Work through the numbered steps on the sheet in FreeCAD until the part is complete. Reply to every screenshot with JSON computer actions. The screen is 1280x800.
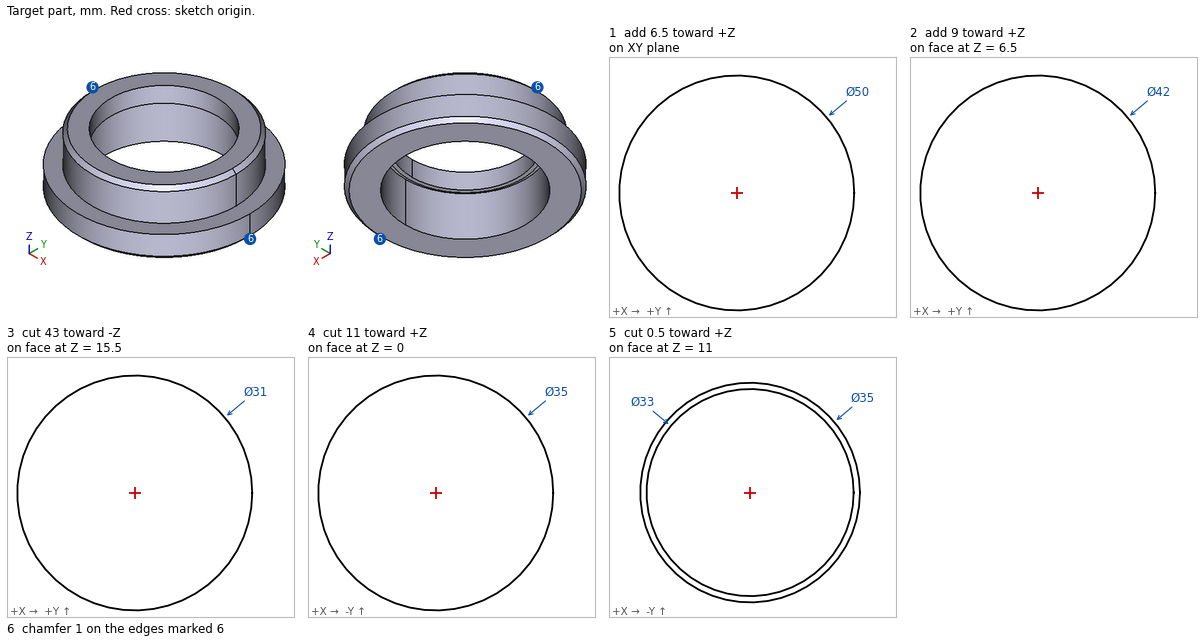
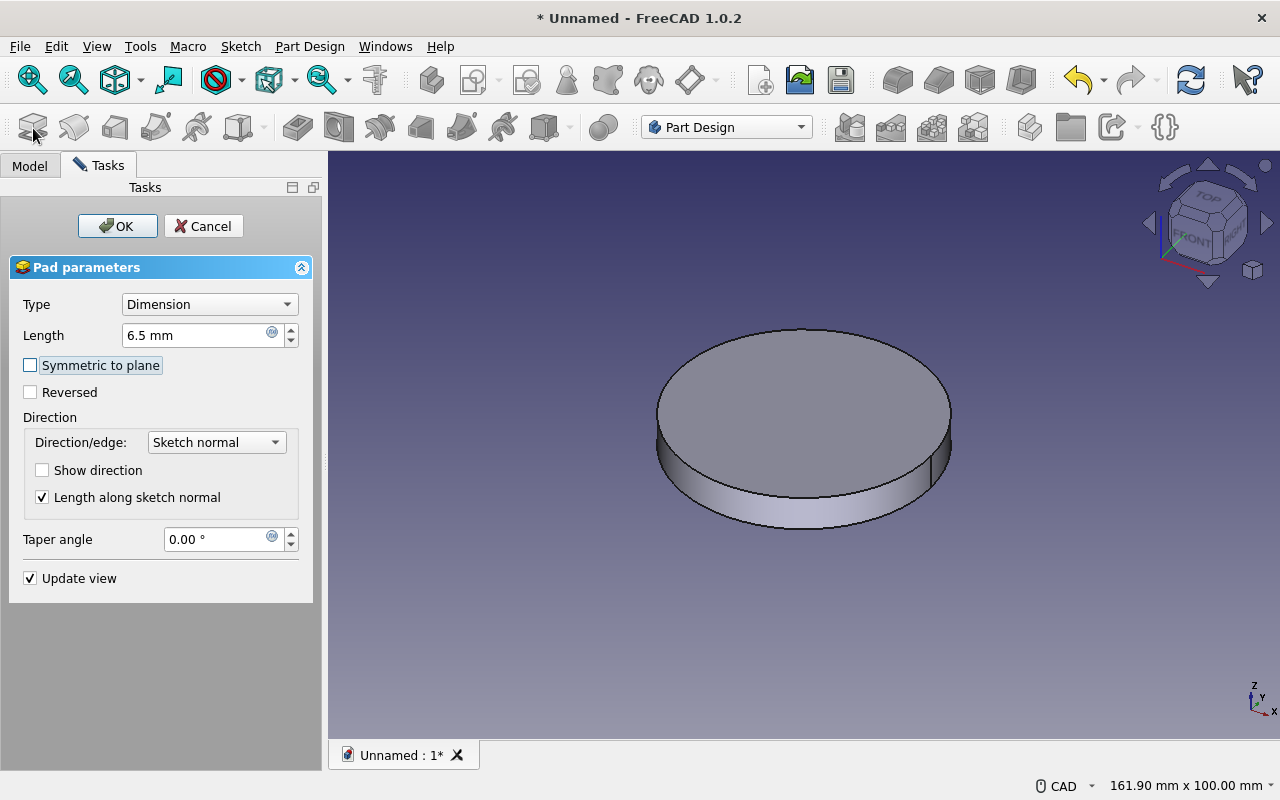
{"action": "left_click", "coordinate": [118, 226]}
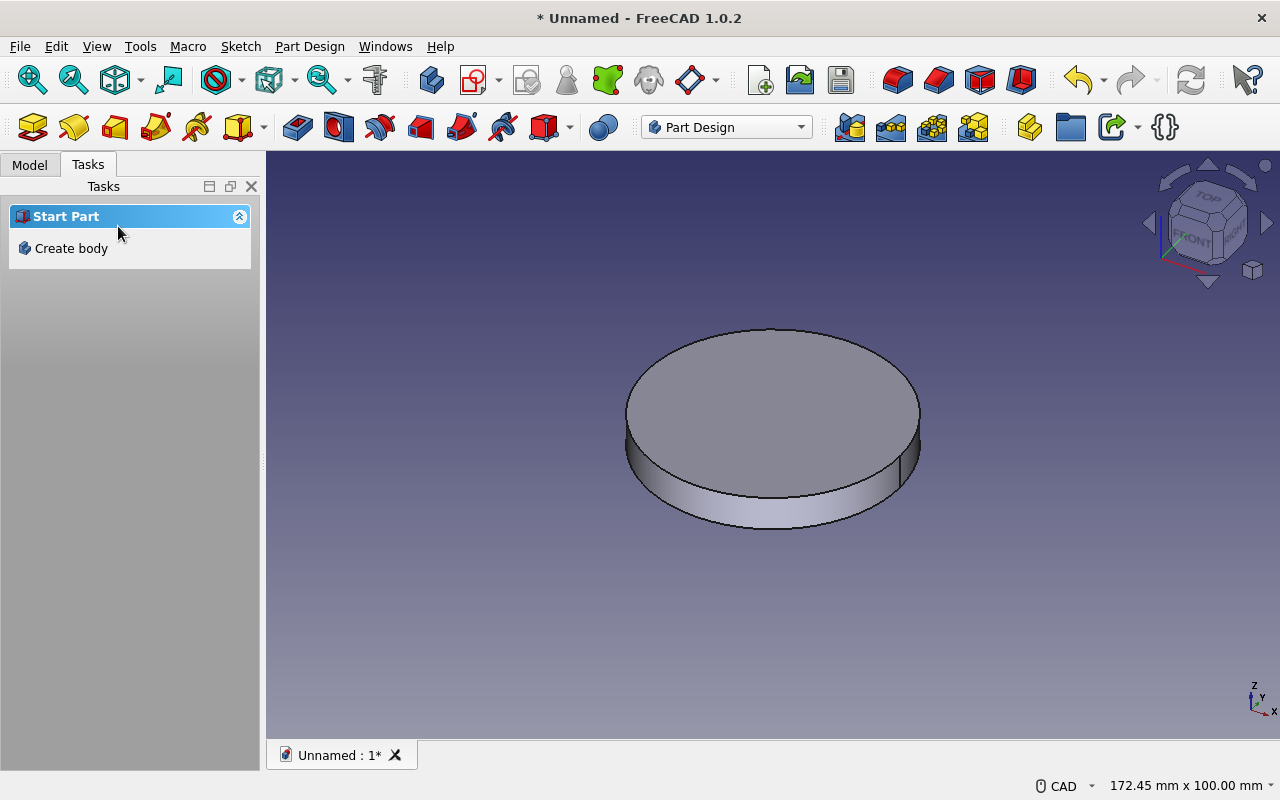
{"action": "left_click", "coordinate": [33, 80]}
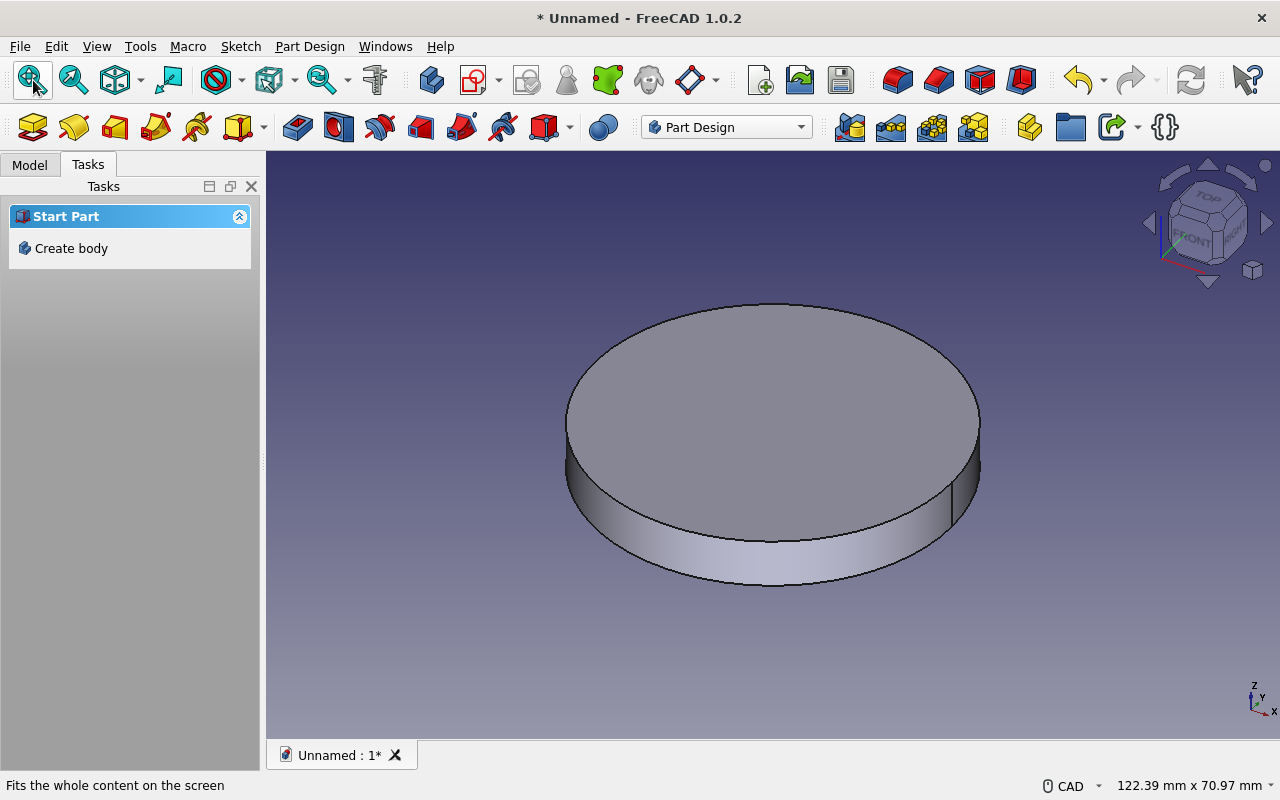
{"action": "left_click", "coordinate": [773, 422]}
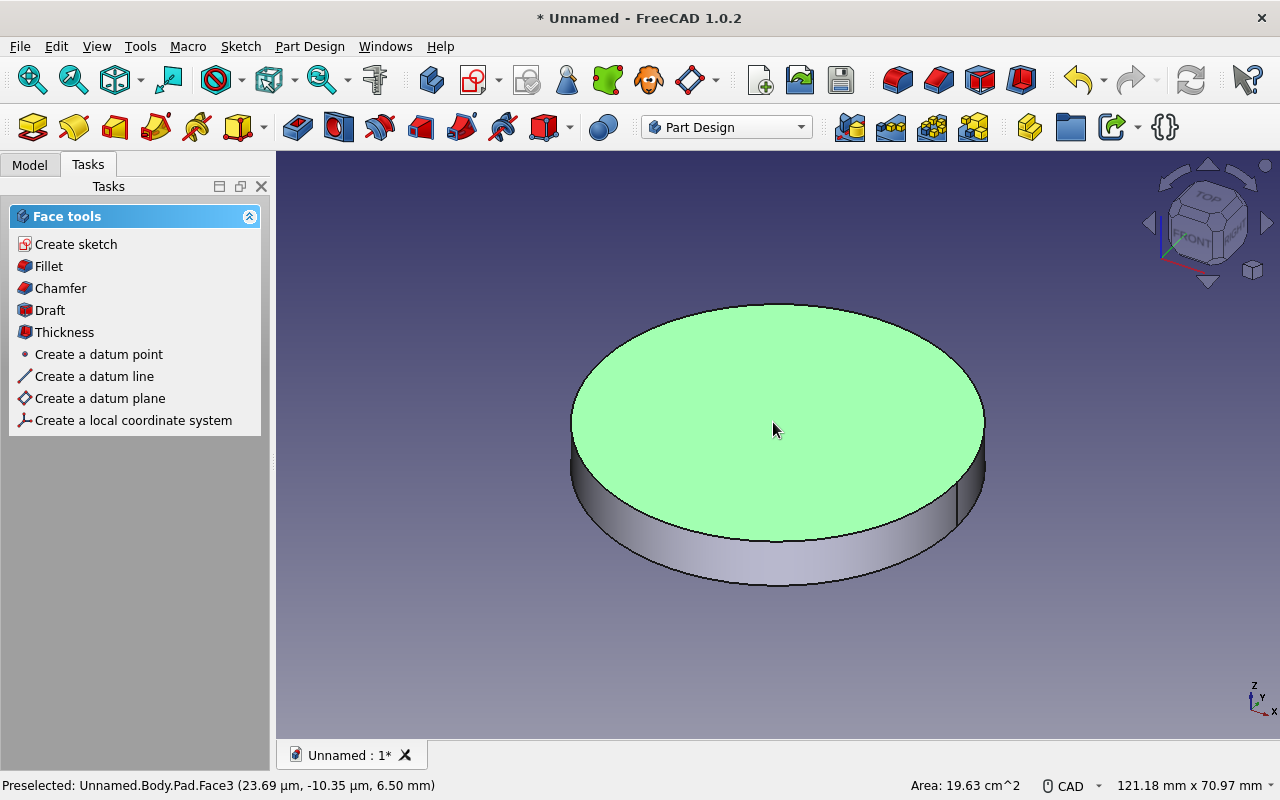
{"action": "left_click", "coordinate": [472, 80]}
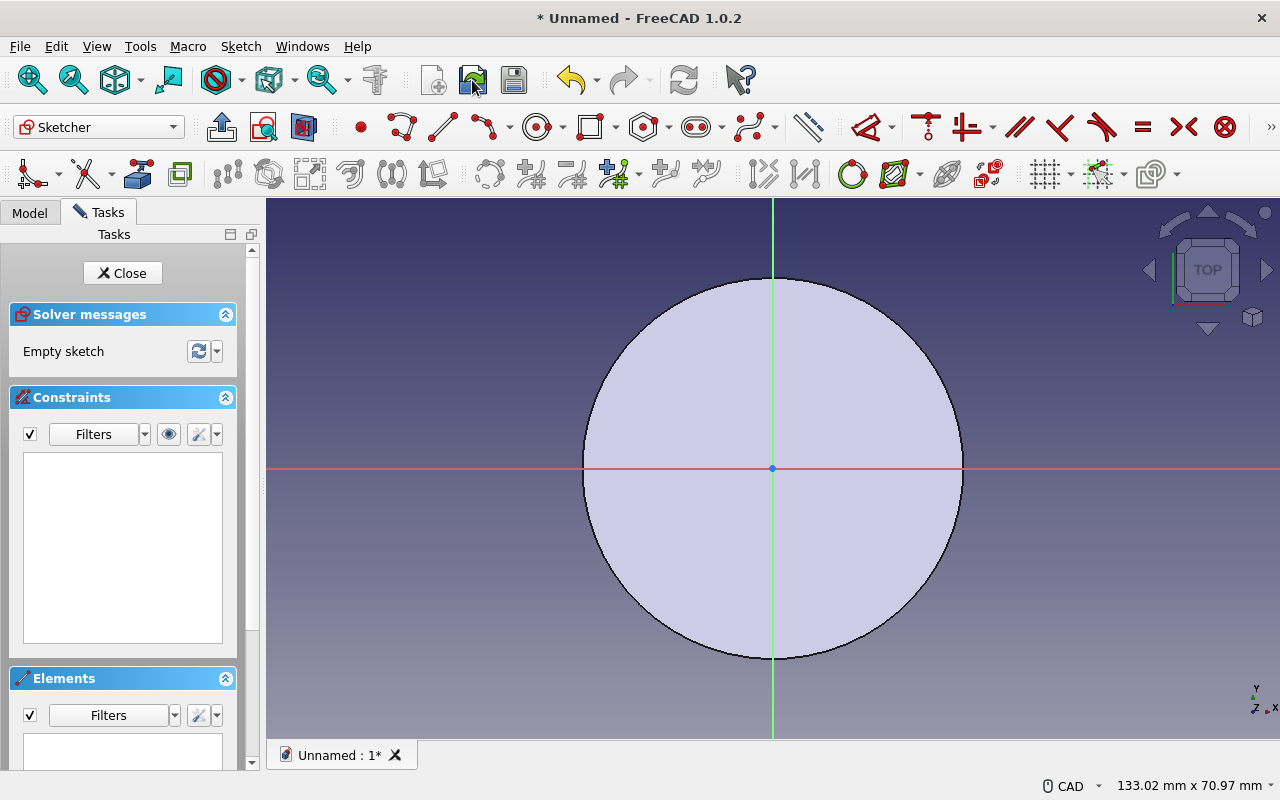
{"action": "left_click", "coordinate": [536, 128]}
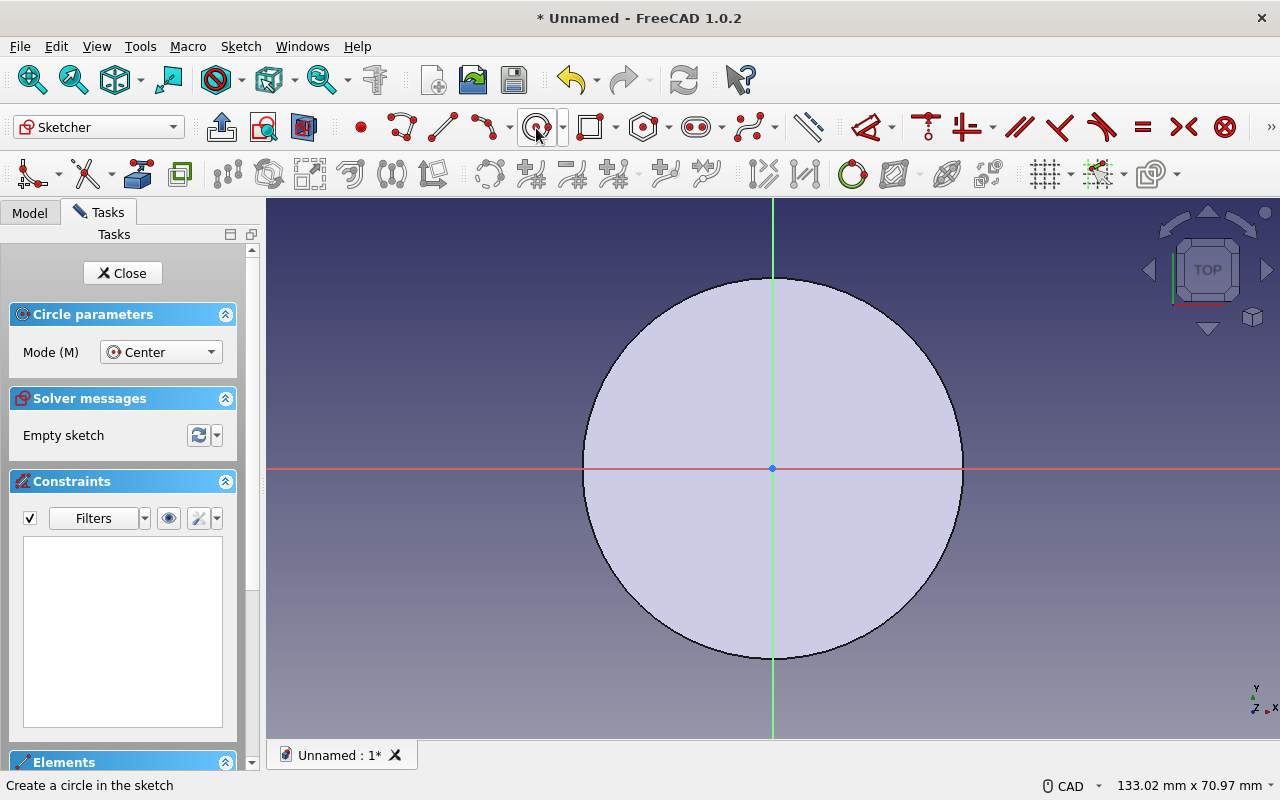
{"action": "left_click", "coordinate": [773, 468]}
{"action": "mouse_move", "coordinate": [886, 355]}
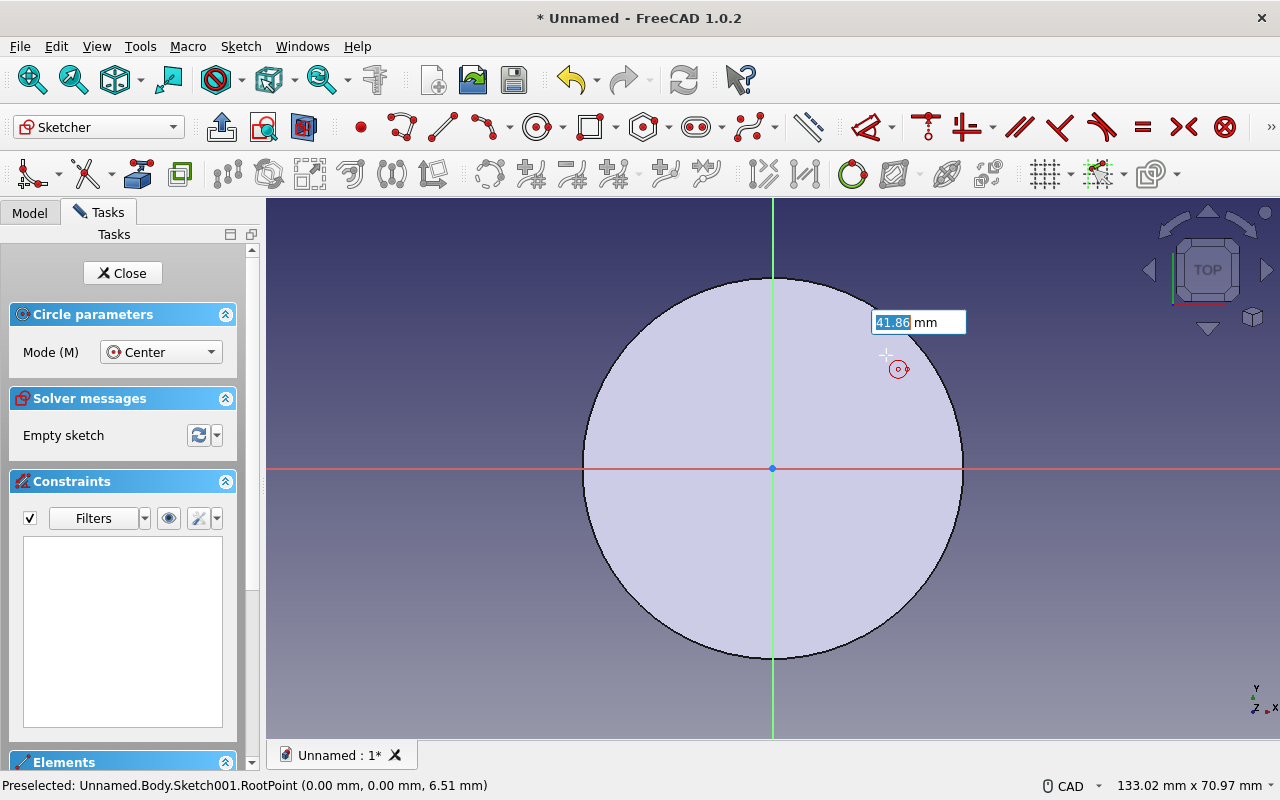
{"action": "type", "text": "42"}
{"action": "key", "text": "Return"}
{"action": "key", "text": "Escape"}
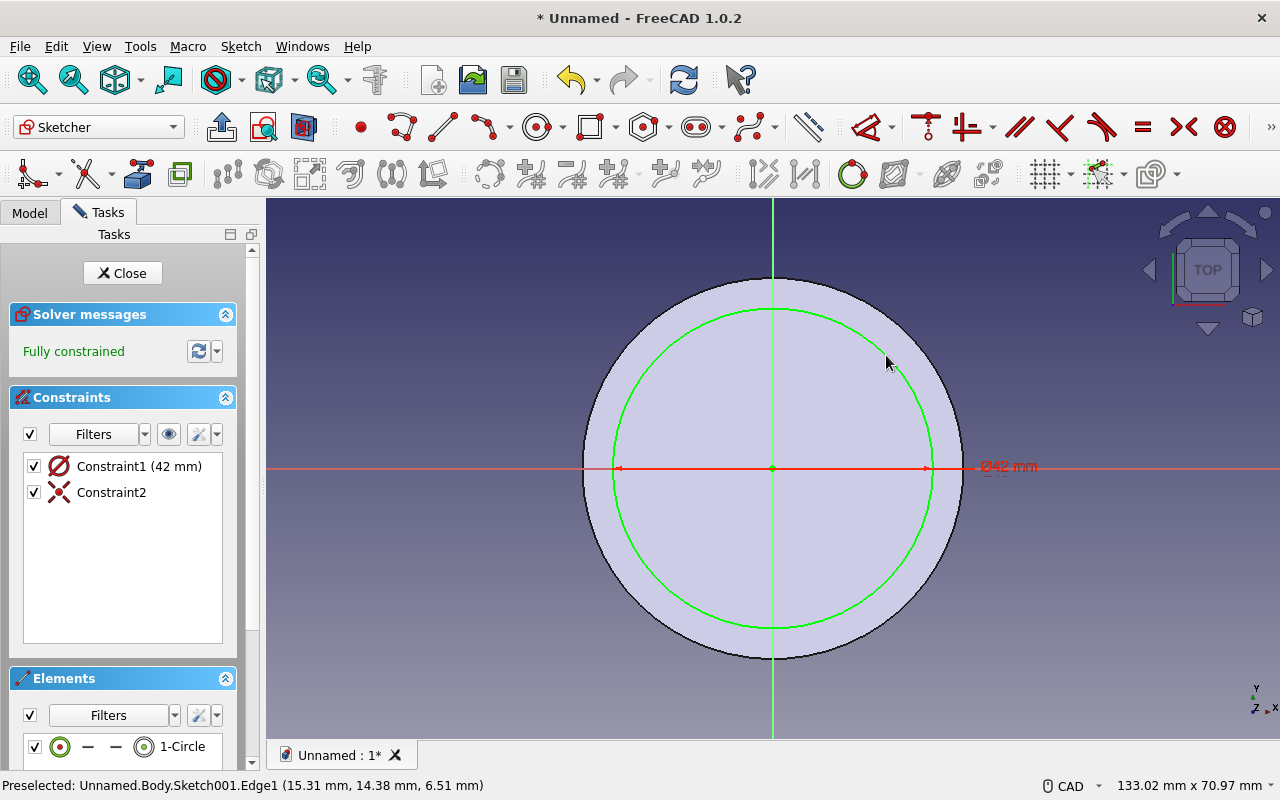
{"action": "left_click", "coordinate": [123, 273]}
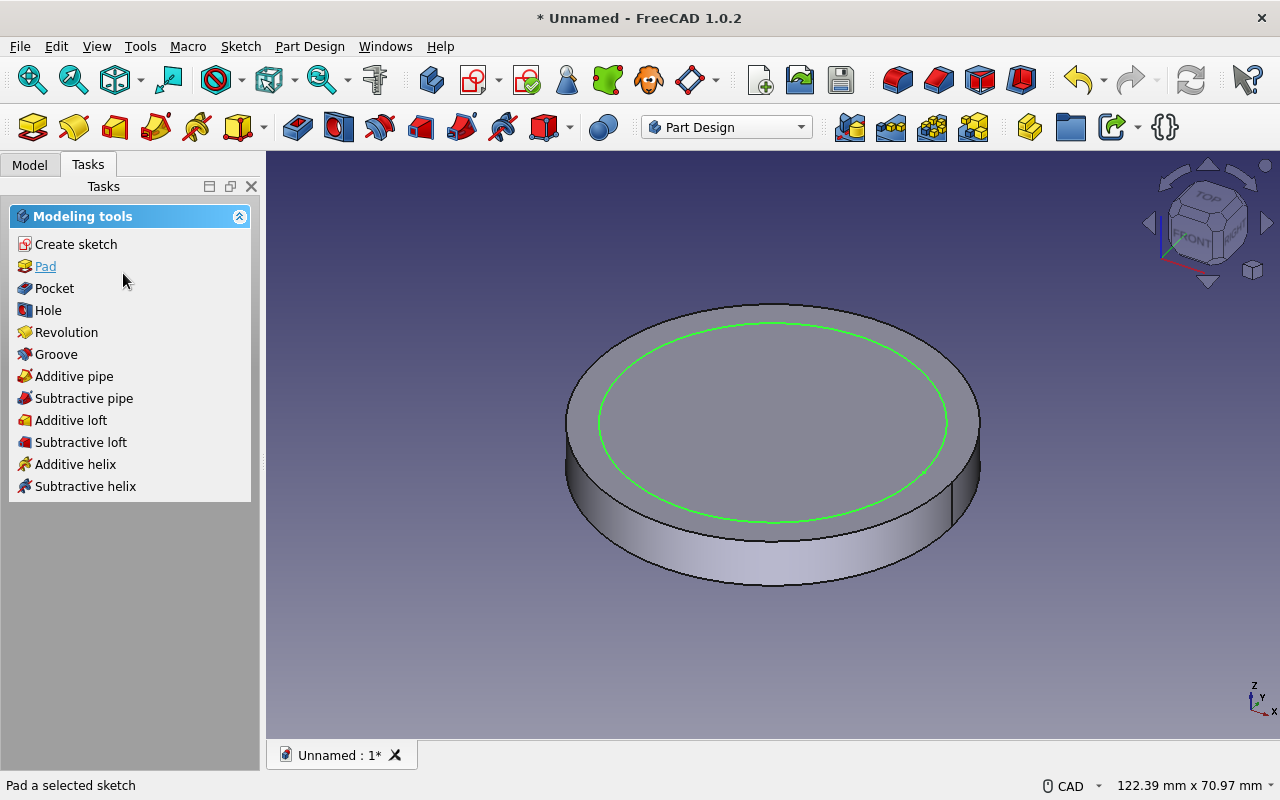
{"action": "left_click", "coordinate": [33, 128]}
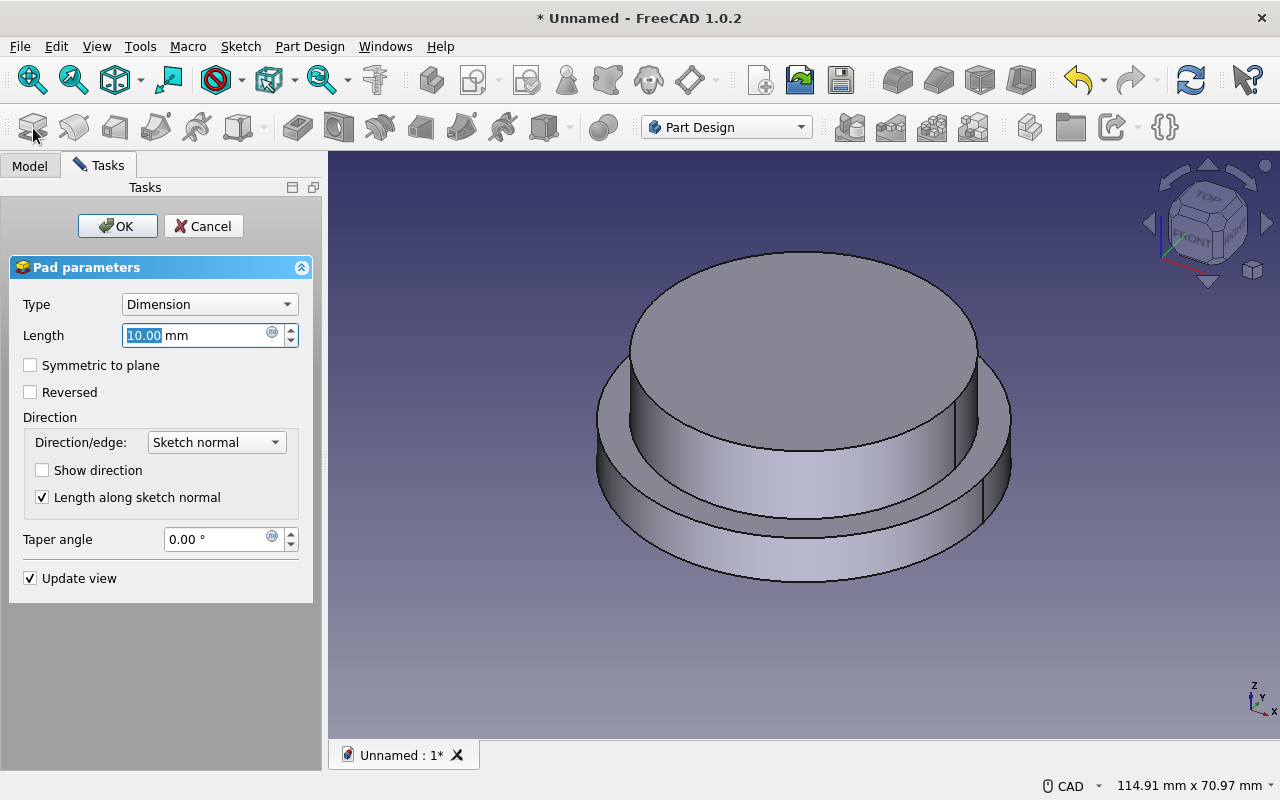
{"action": "type", "text": "9"}
{"action": "key", "text": "Tab"}